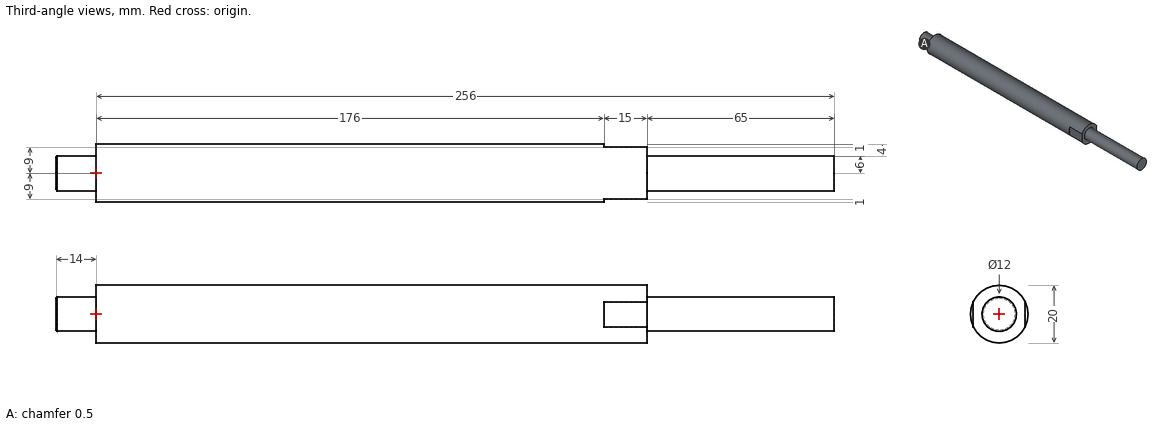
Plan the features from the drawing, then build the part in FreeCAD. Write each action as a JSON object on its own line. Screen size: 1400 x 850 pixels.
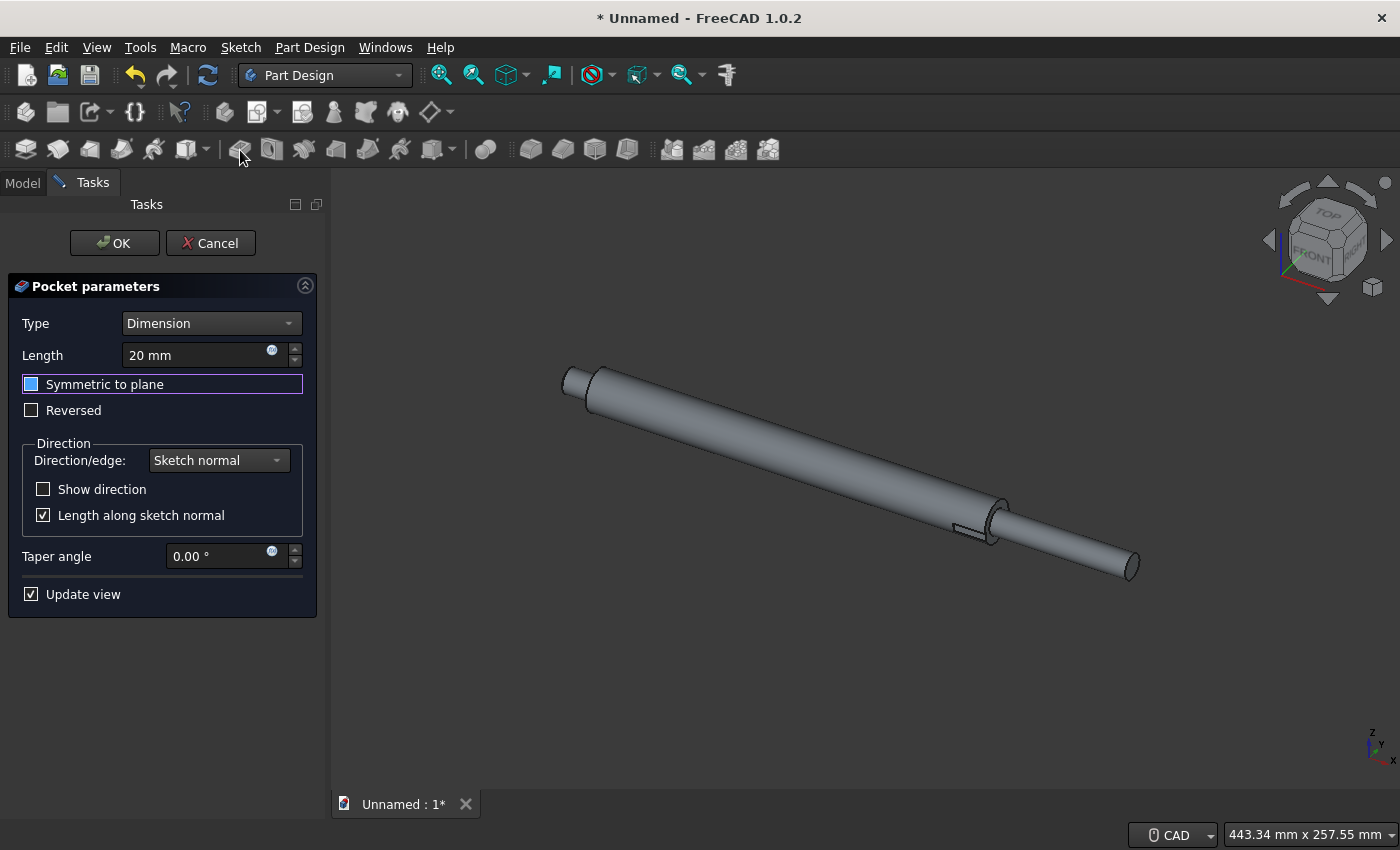
{"action": "left_click", "coordinate": [30, 384]}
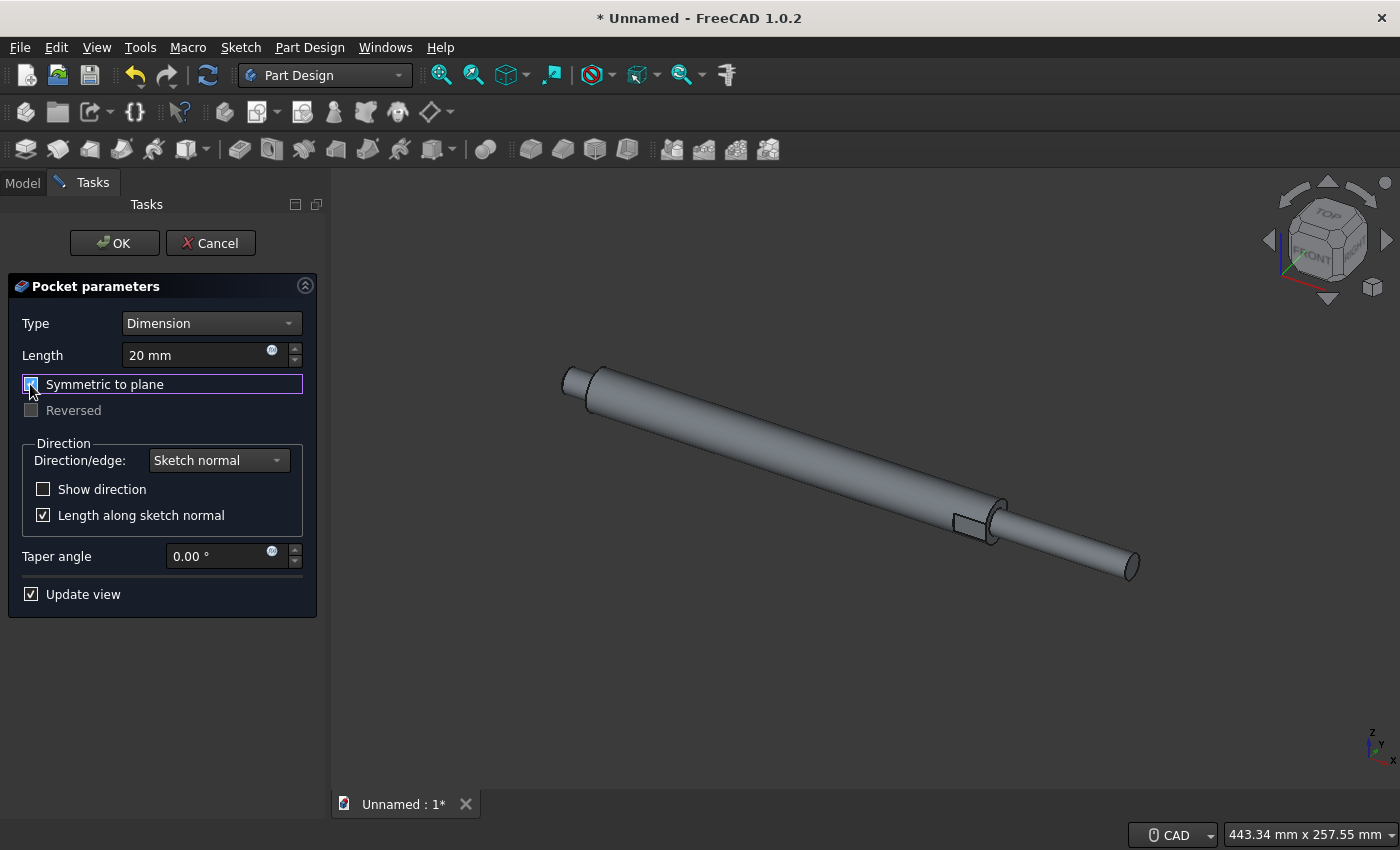
{"action": "left_click", "coordinate": [115, 243]}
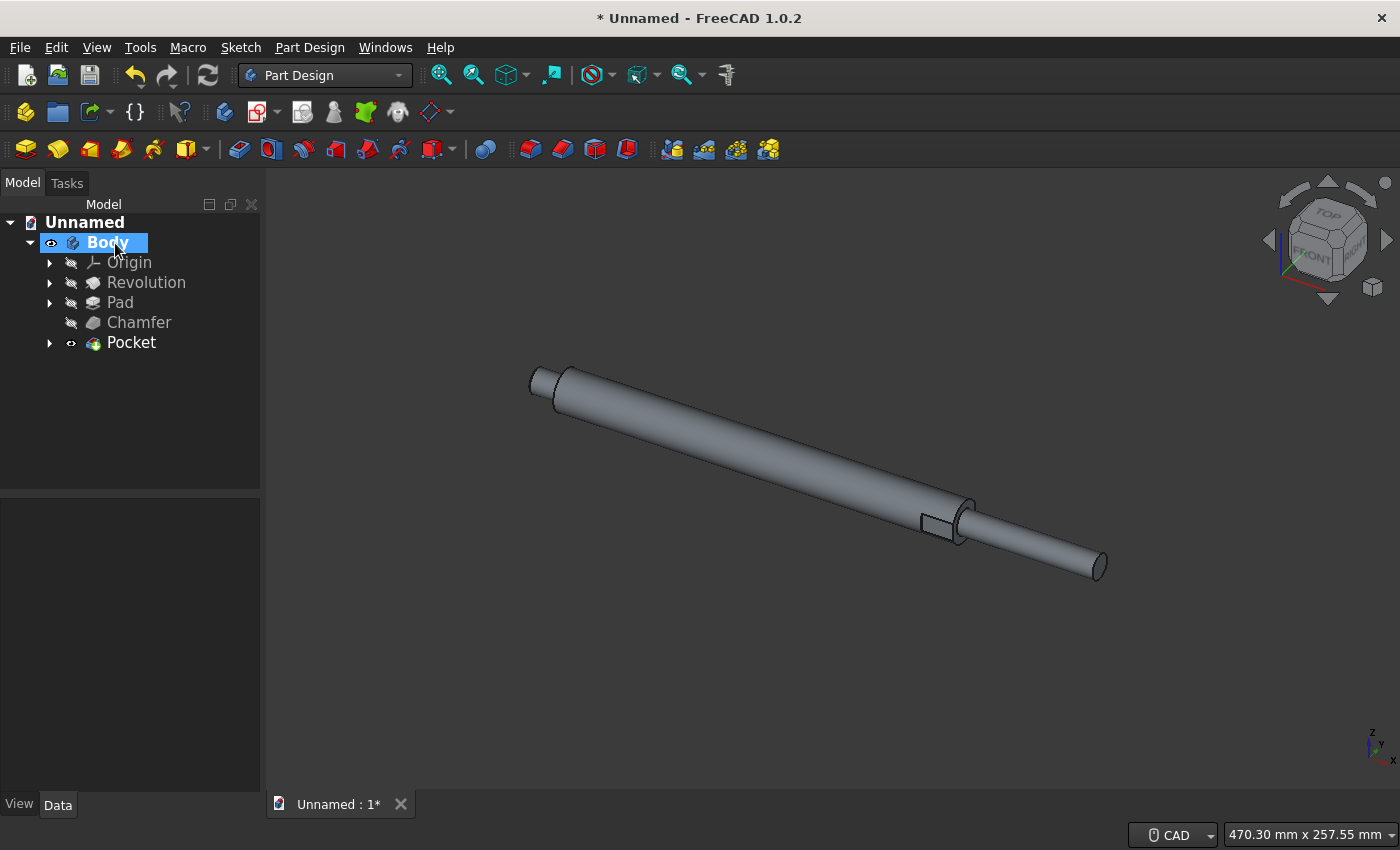
{"action": "key", "text": "0"}